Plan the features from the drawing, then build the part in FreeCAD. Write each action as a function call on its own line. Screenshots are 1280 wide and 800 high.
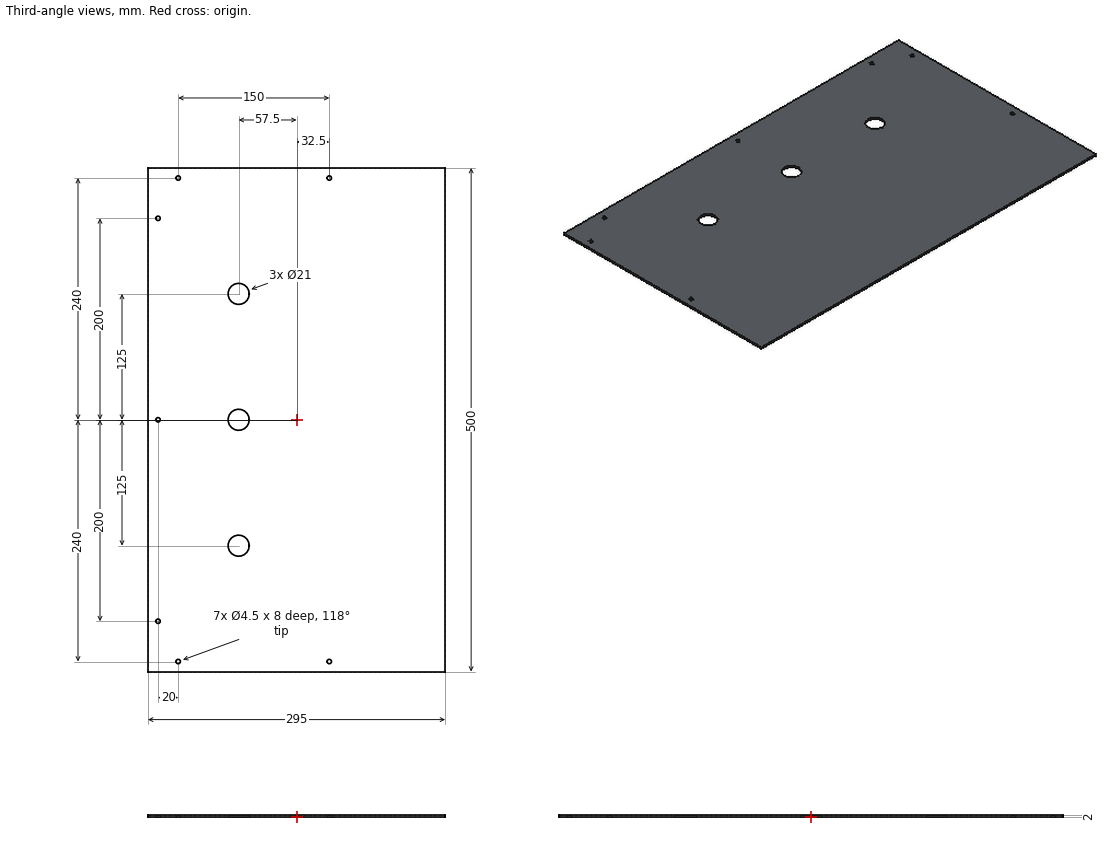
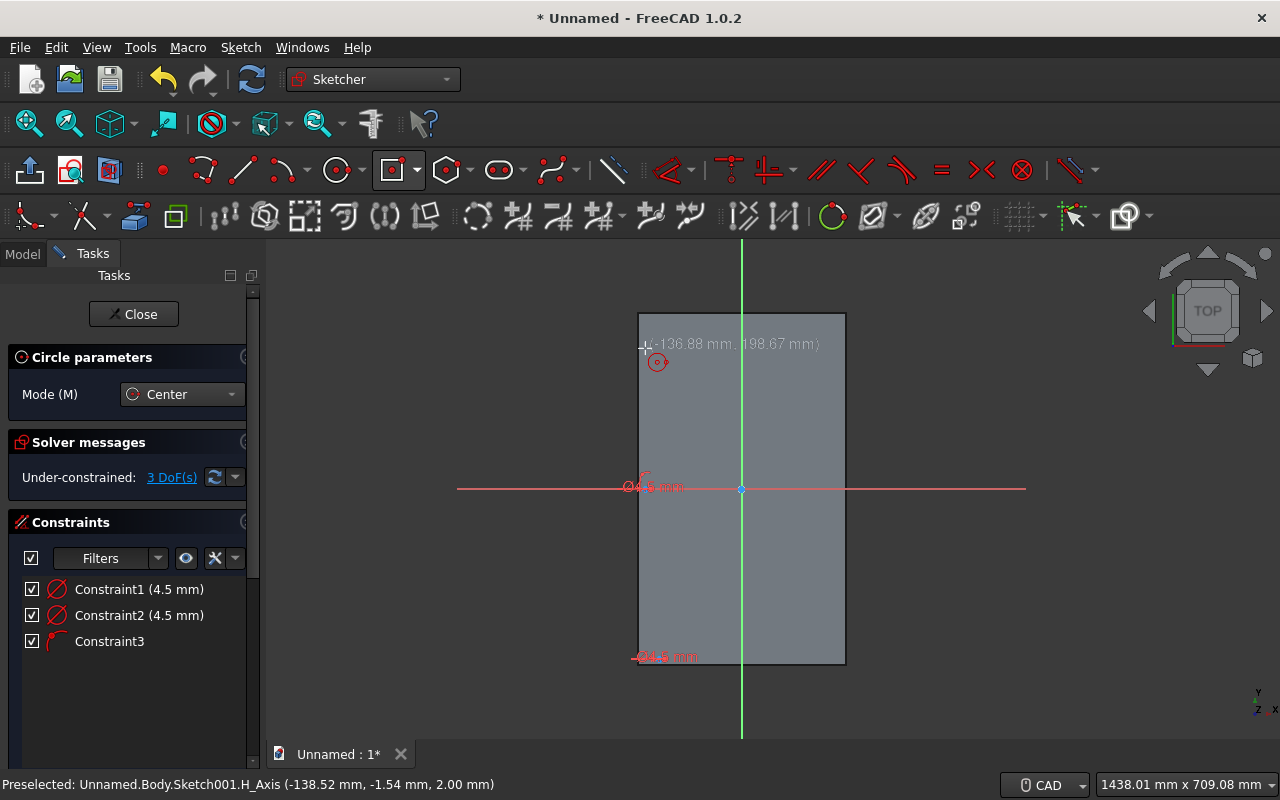
click(645, 348)
move(646, 347)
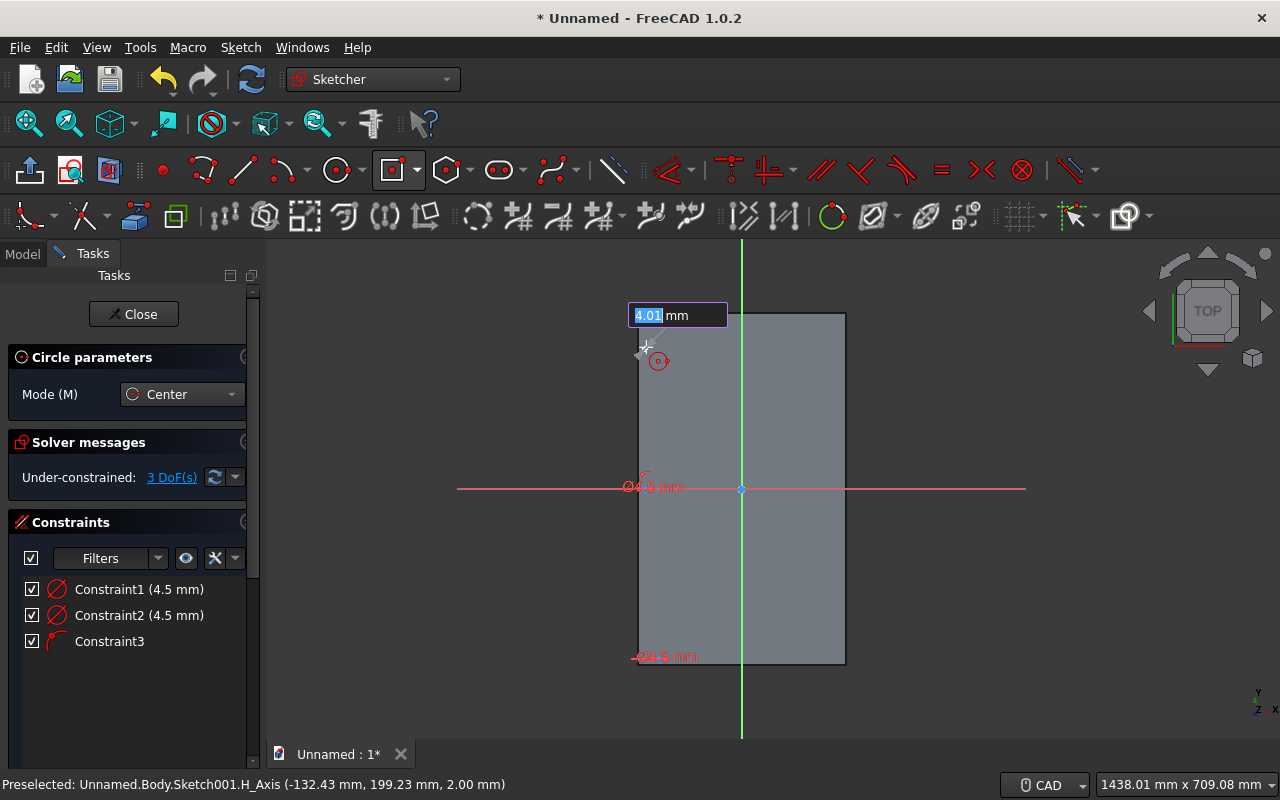
text(4.5)
key(Return)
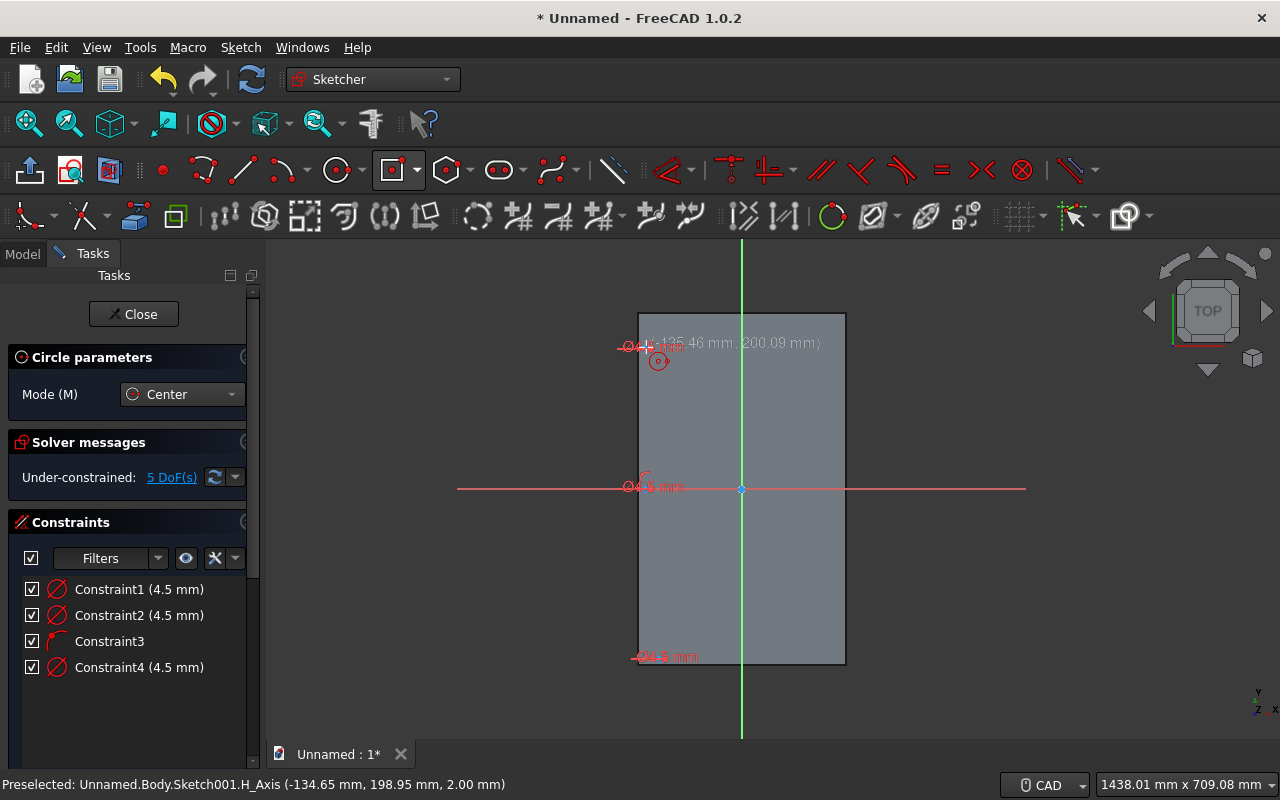
scroll(645, 630, up, 14)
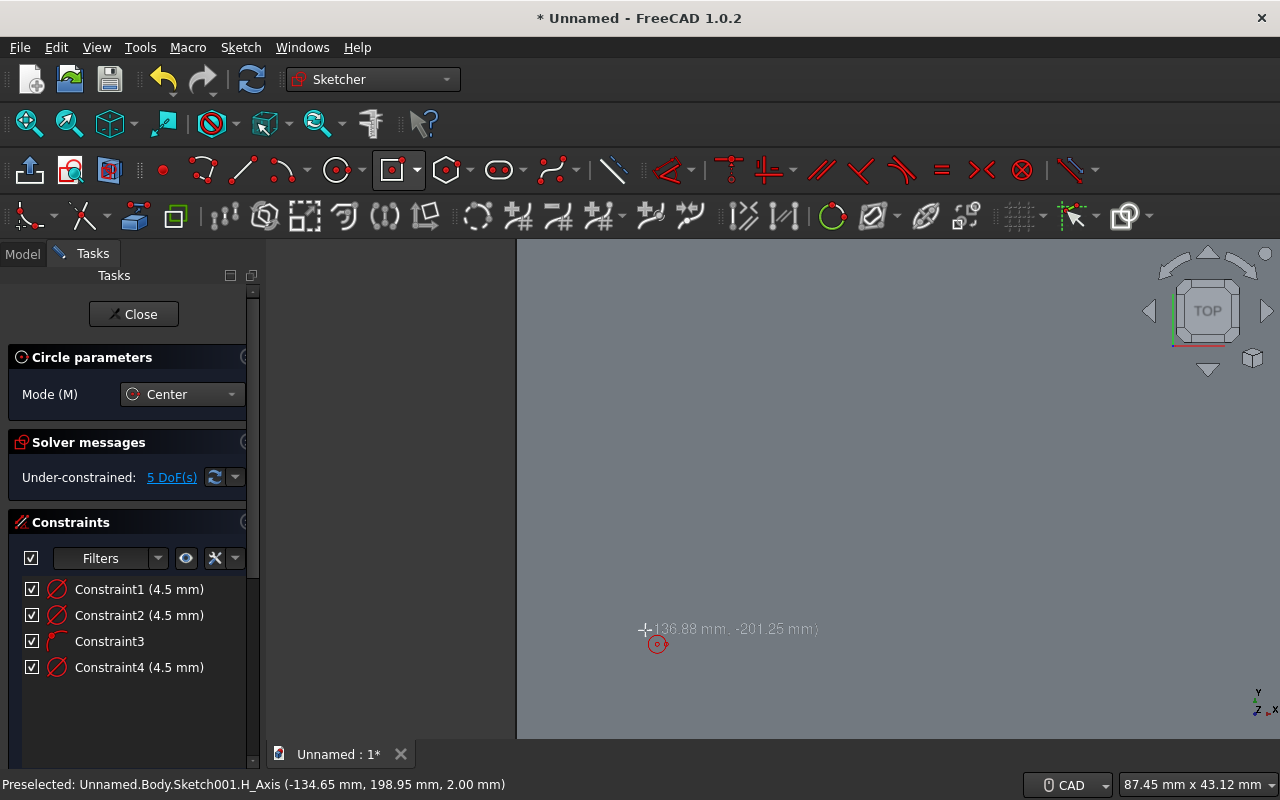
scroll(645, 631, down, 14)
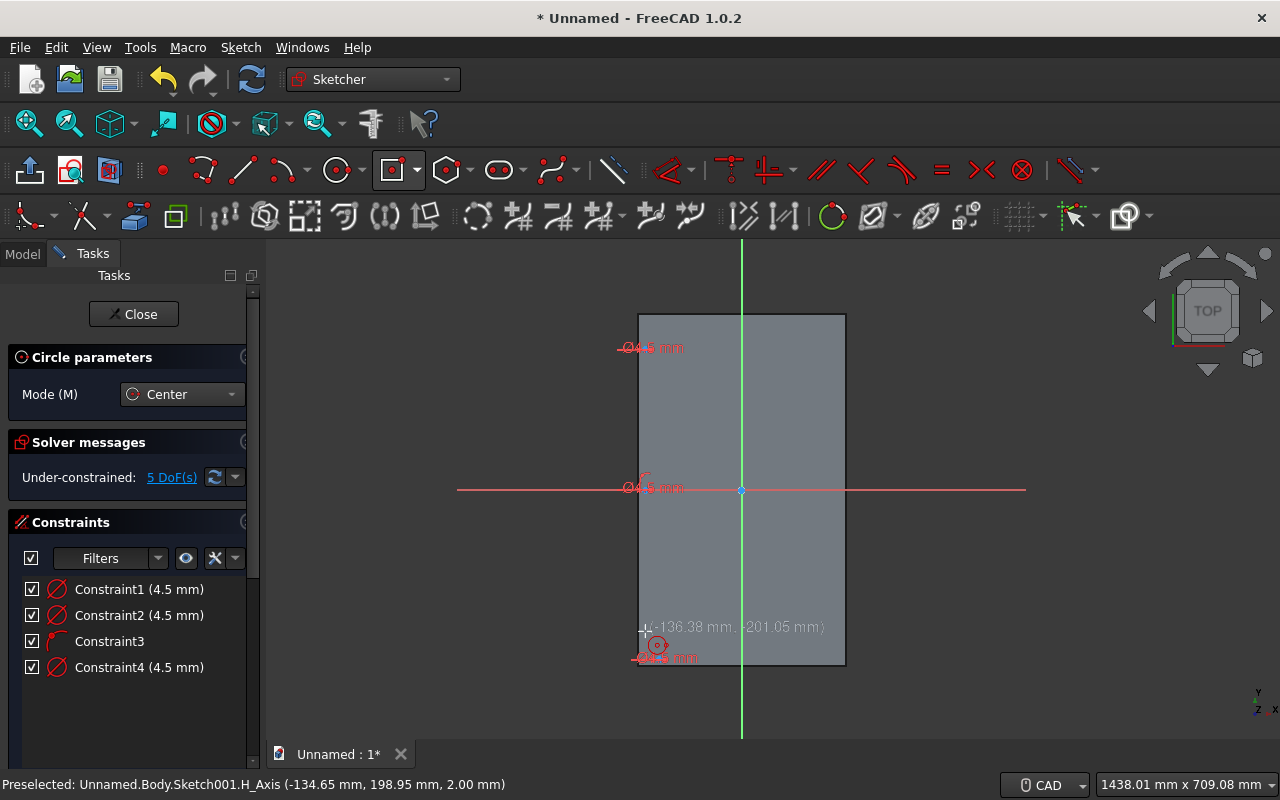
click(645, 631)
move(646, 630)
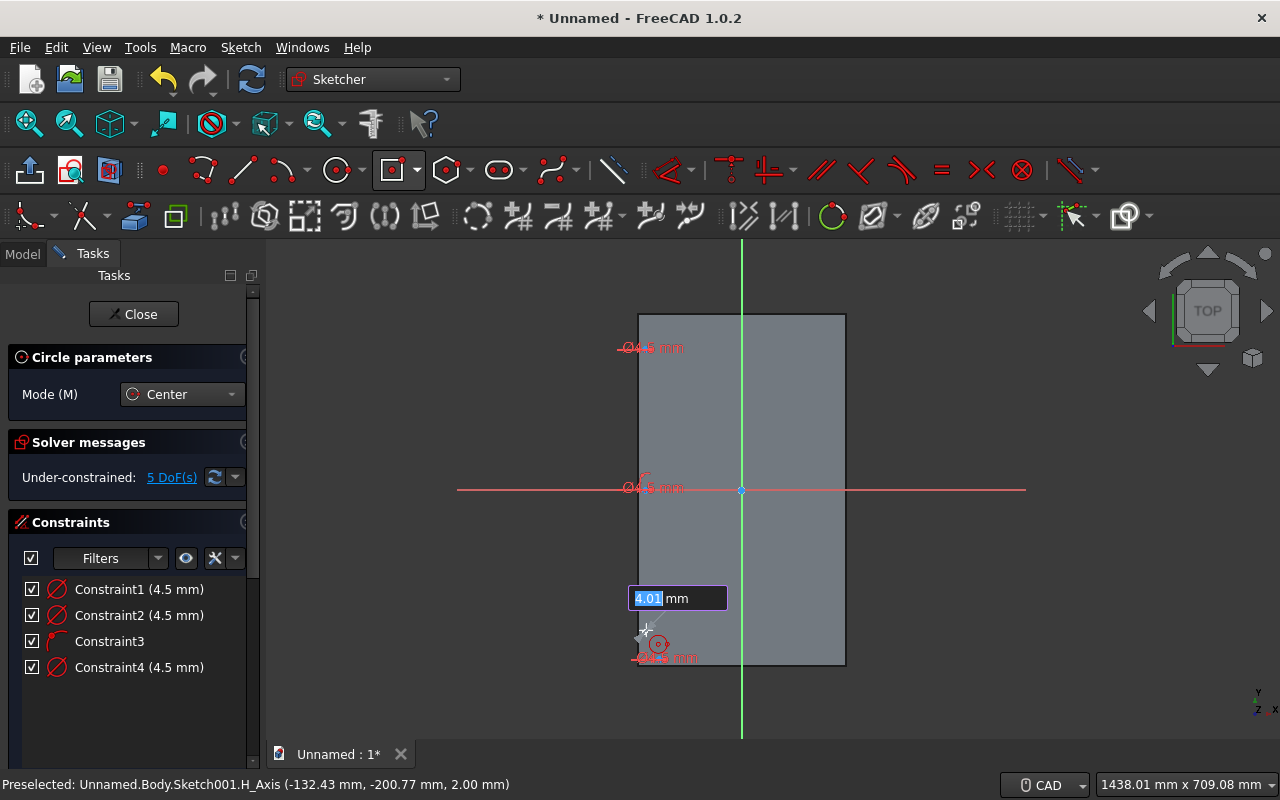
text(4.5)
key(Return)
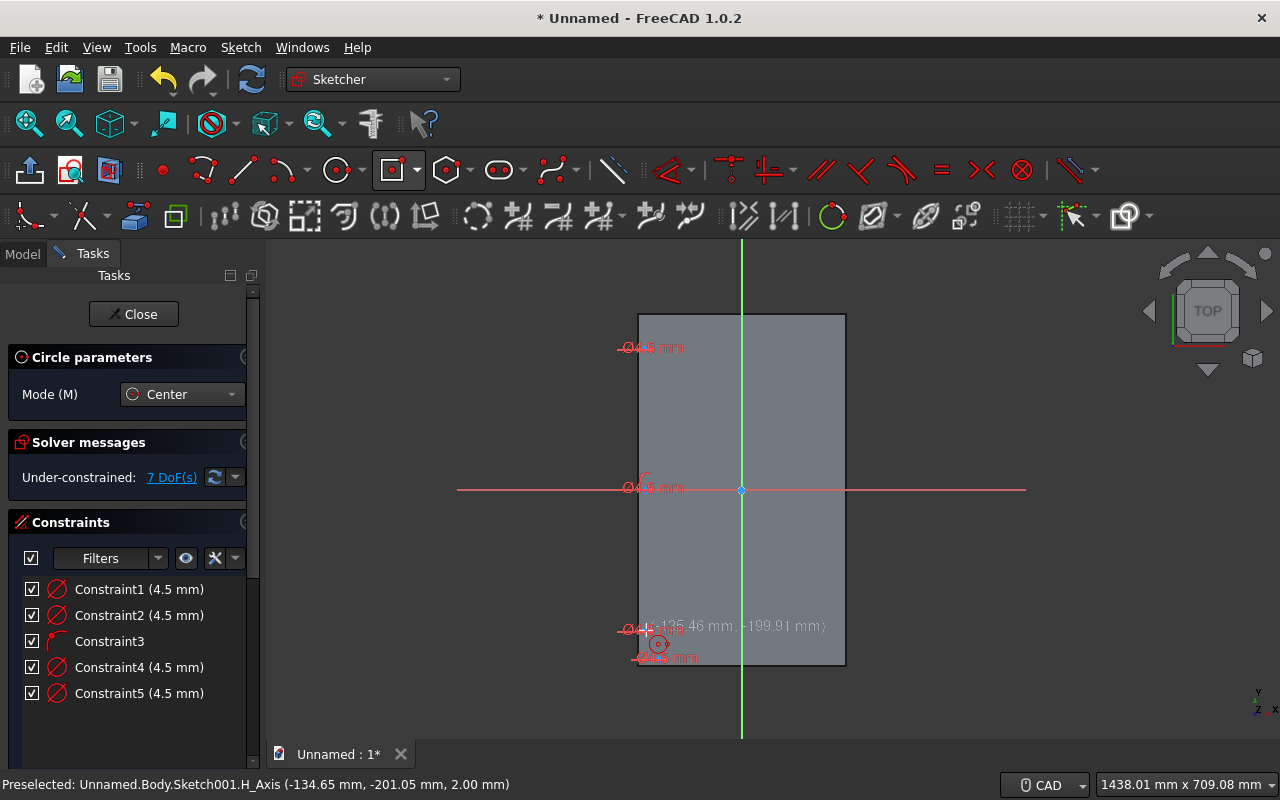
scroll(659, 321, up, 14)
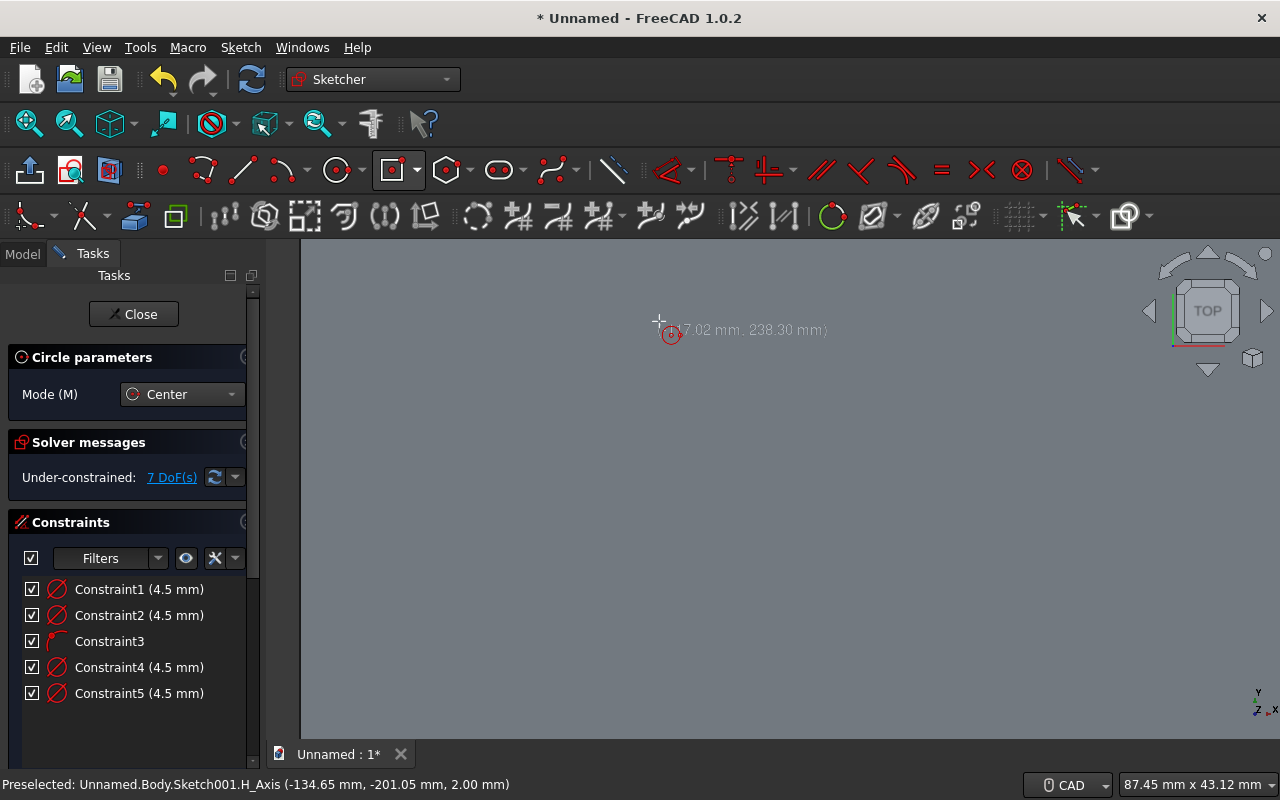
scroll(659, 320, down, 14)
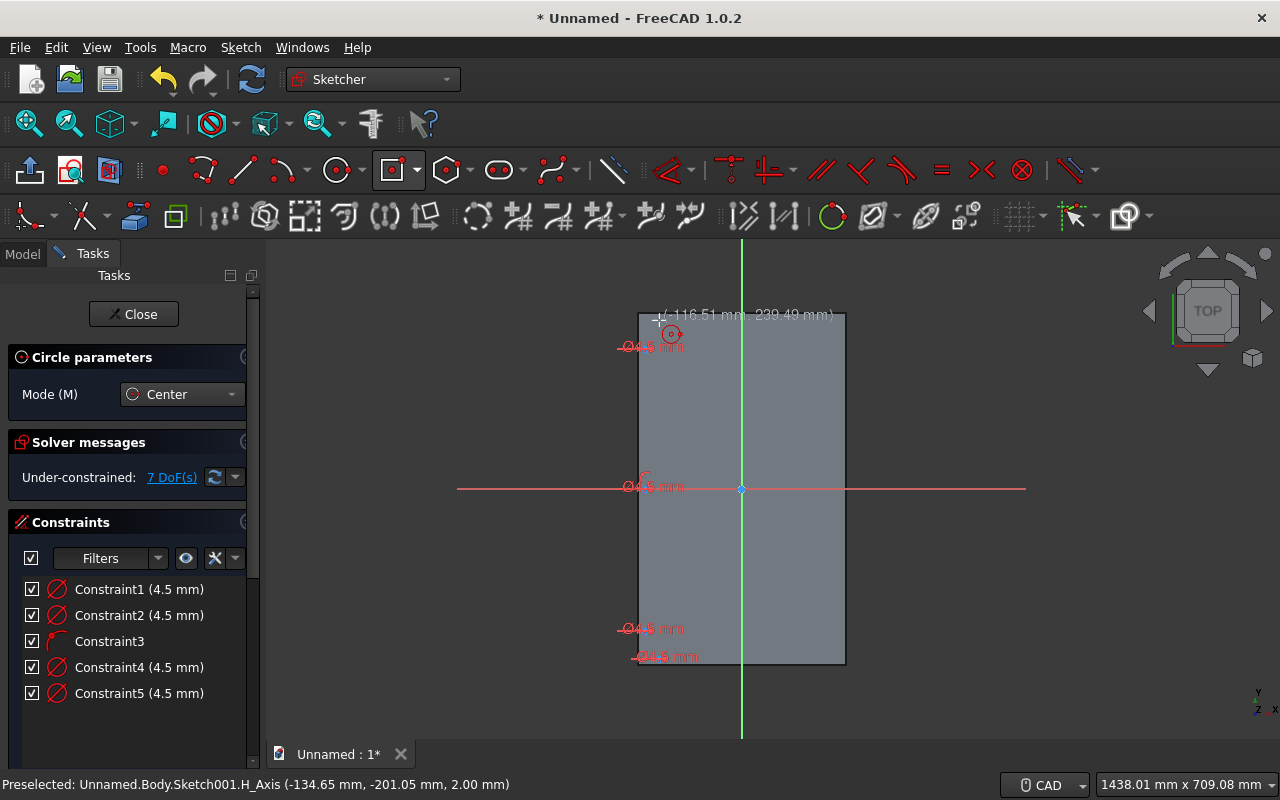
click(659, 320)
move(660, 319)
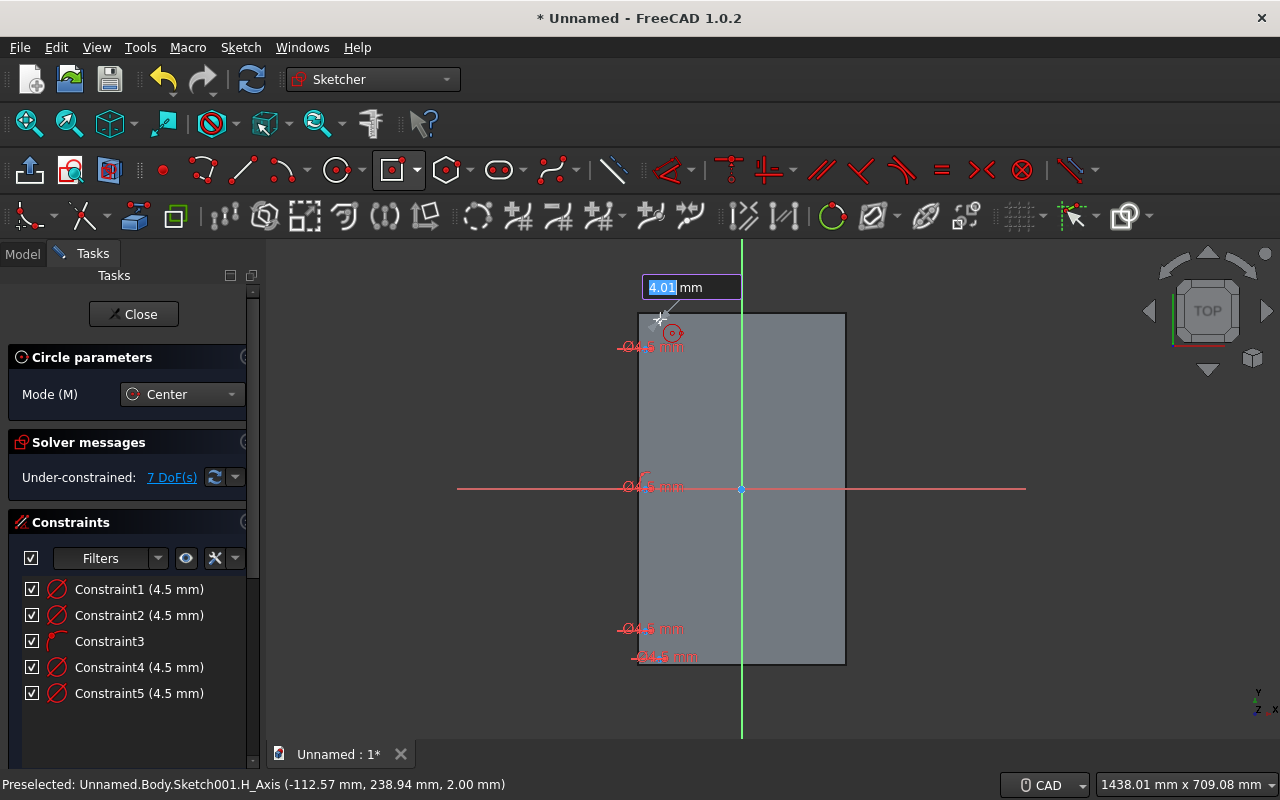
text(4.5)
key(Return)